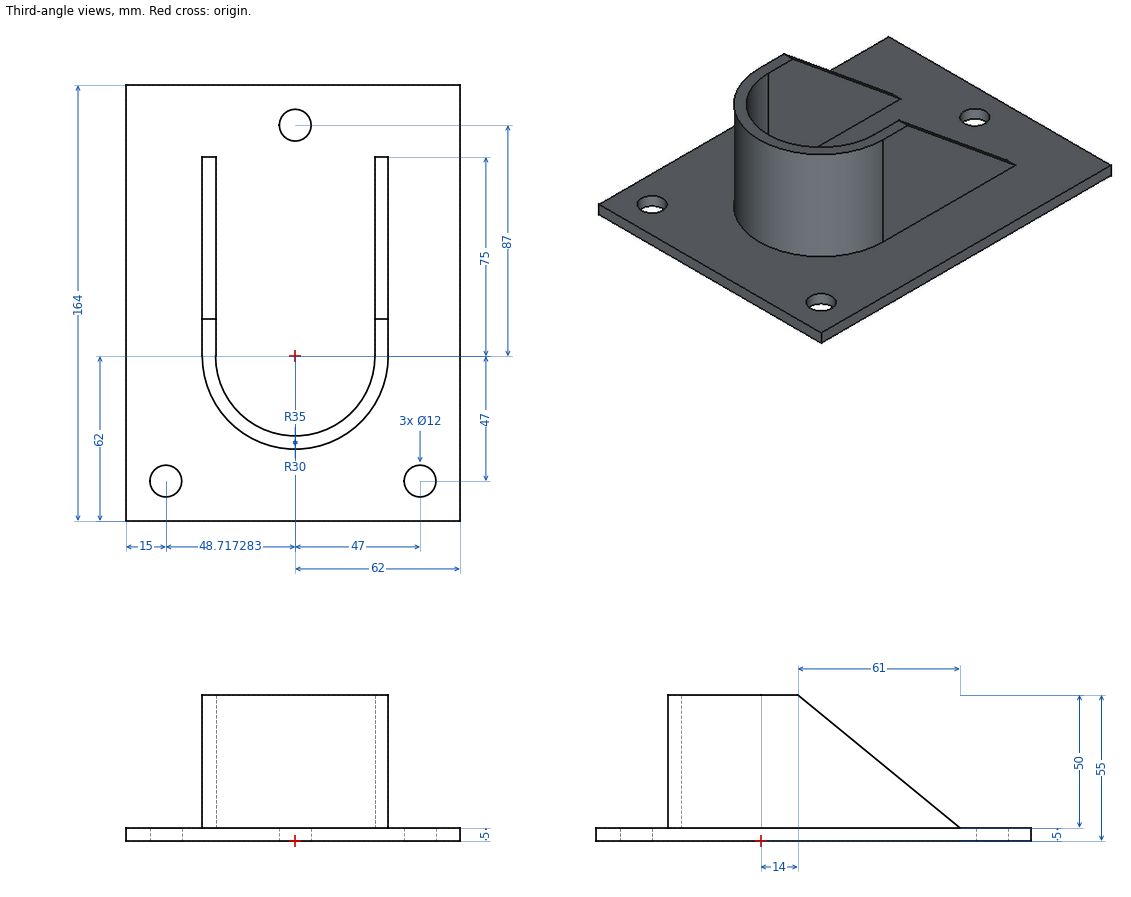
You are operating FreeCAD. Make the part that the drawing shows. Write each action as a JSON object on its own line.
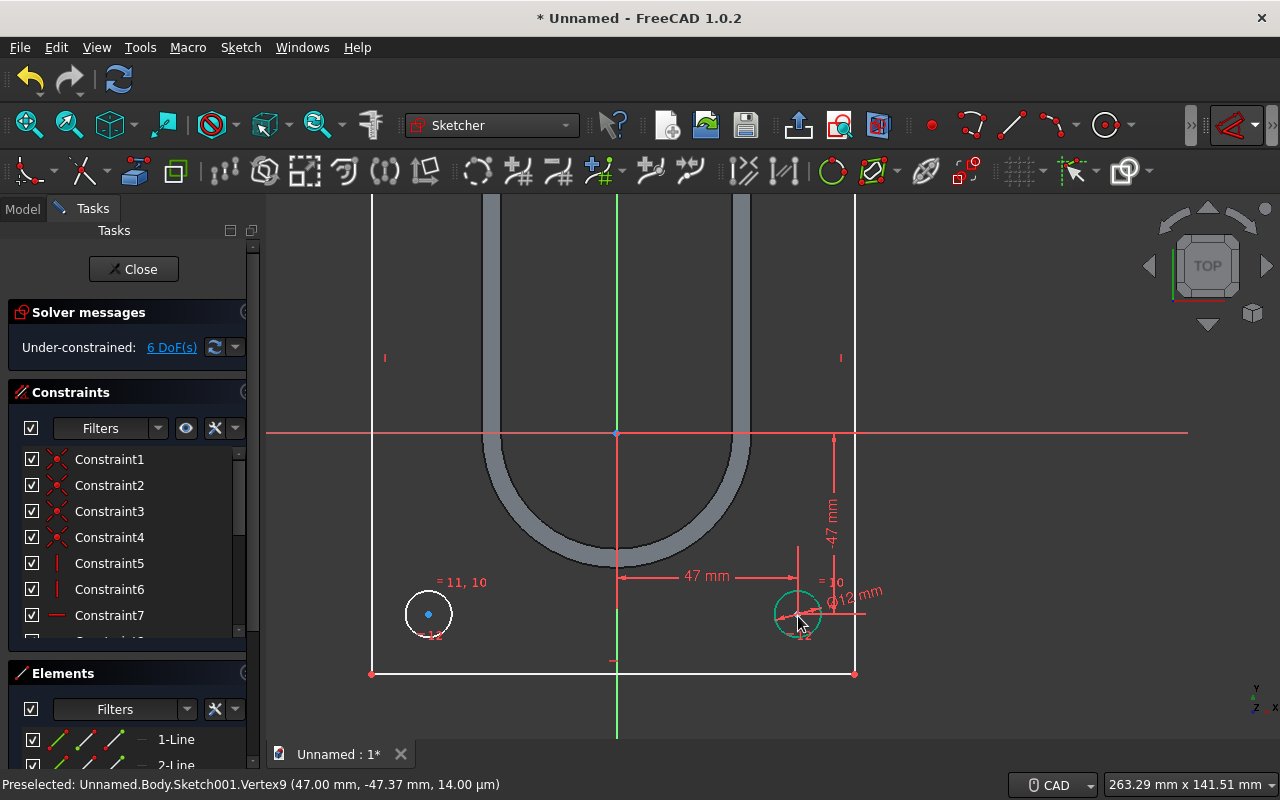
{"action": "scroll", "coordinate": [815, 601], "scroll_direction": "down", "scroll_amount": 3}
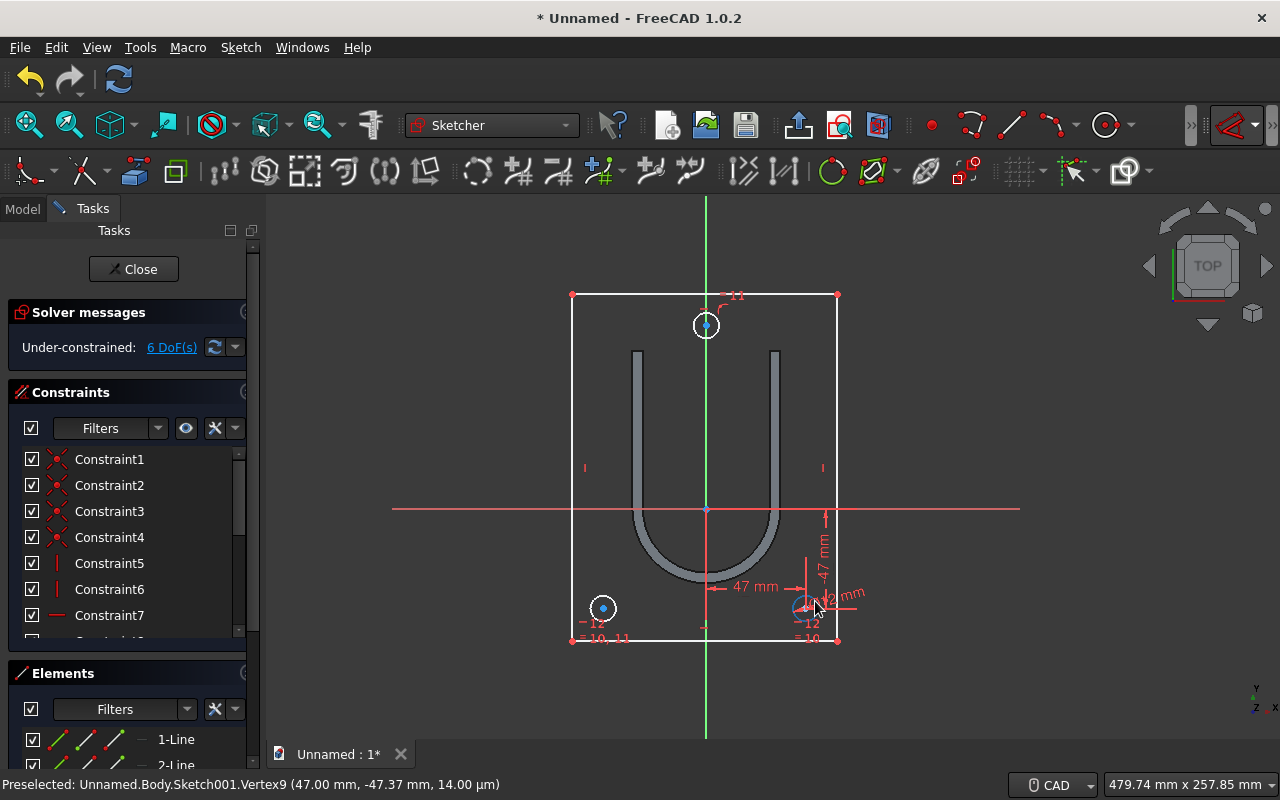
{"action": "left_click", "coordinate": [706, 326]}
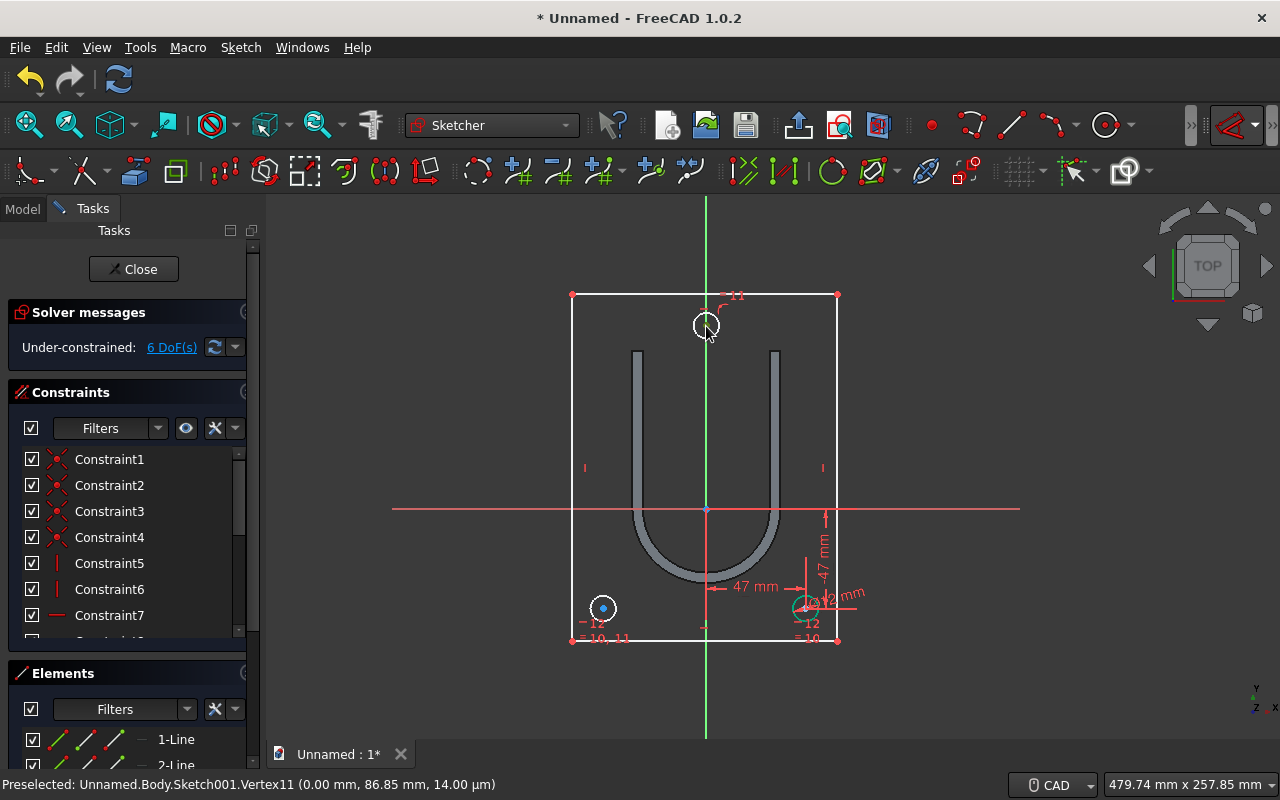
{"action": "left_click", "coordinate": [1258, 126]}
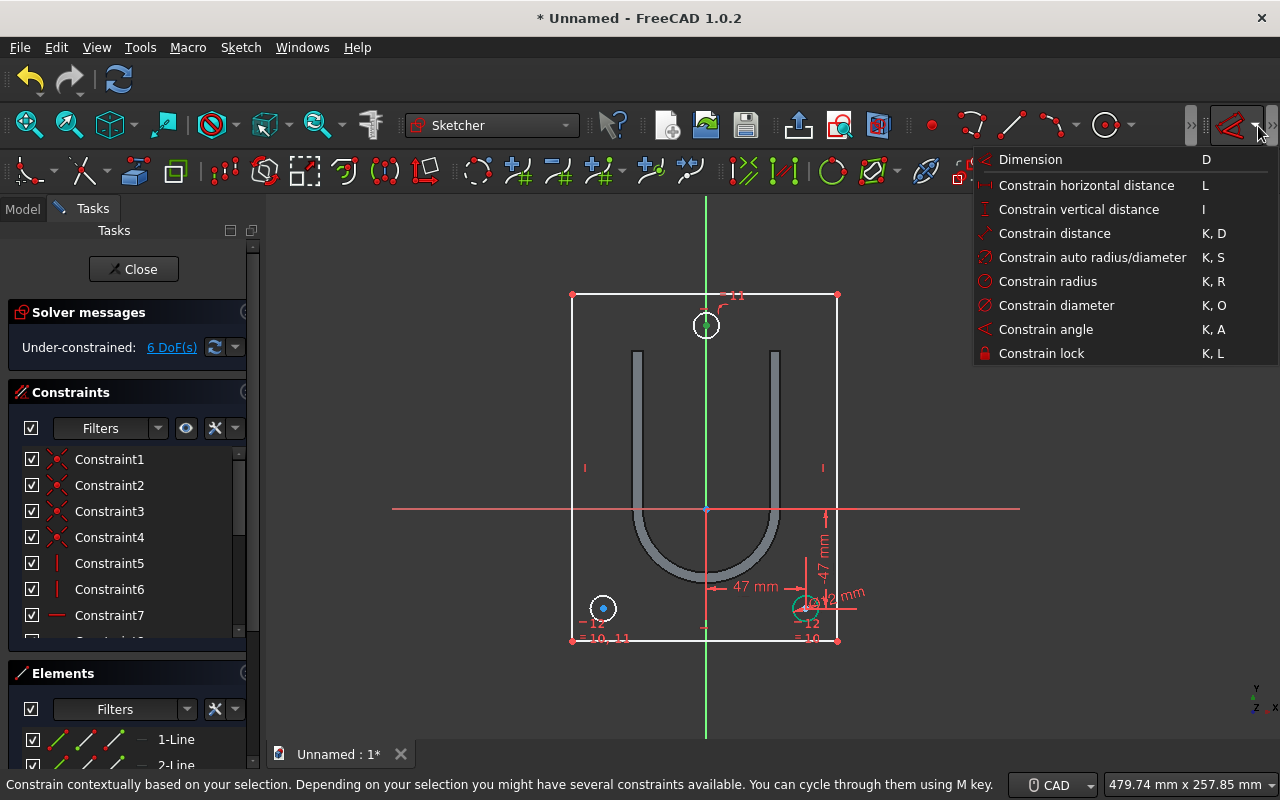
{"action": "left_click", "coordinate": [1126, 209]}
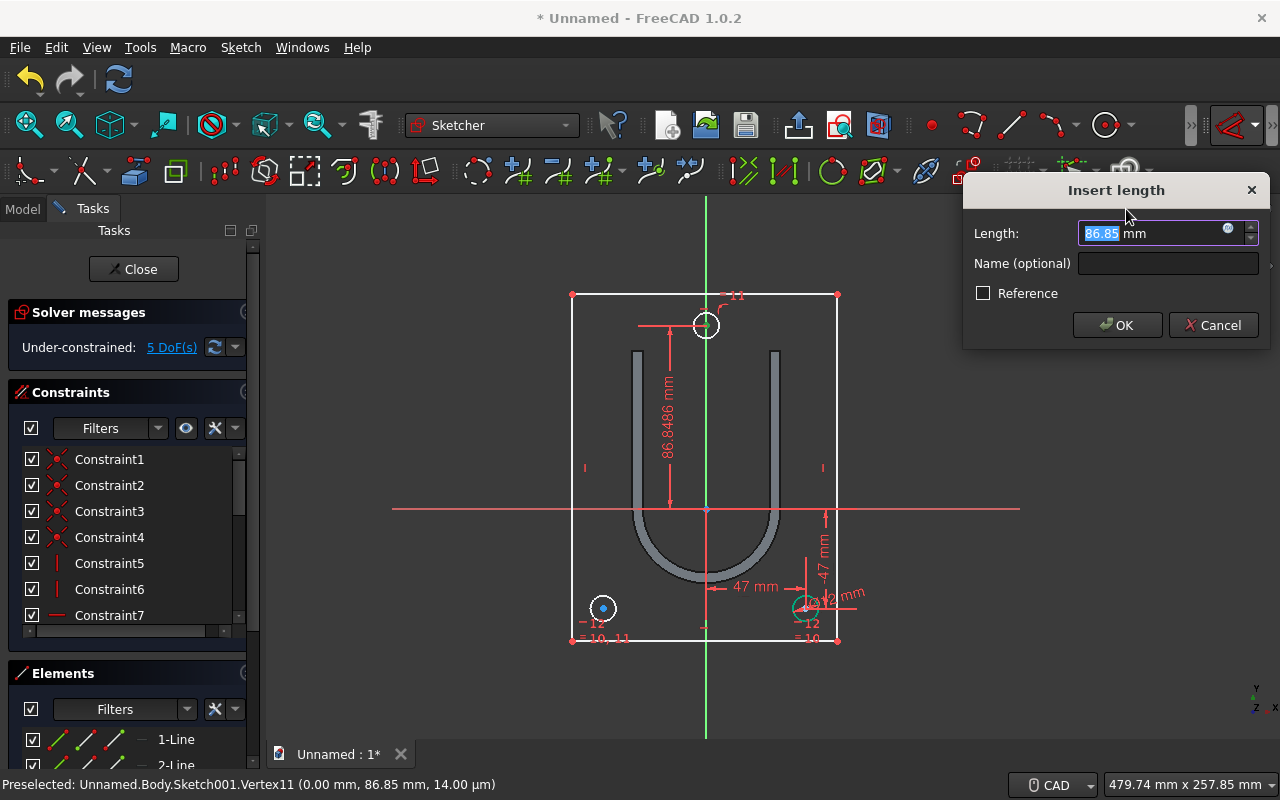
{"action": "type", "text": "87"}
{"action": "key", "text": "Return"}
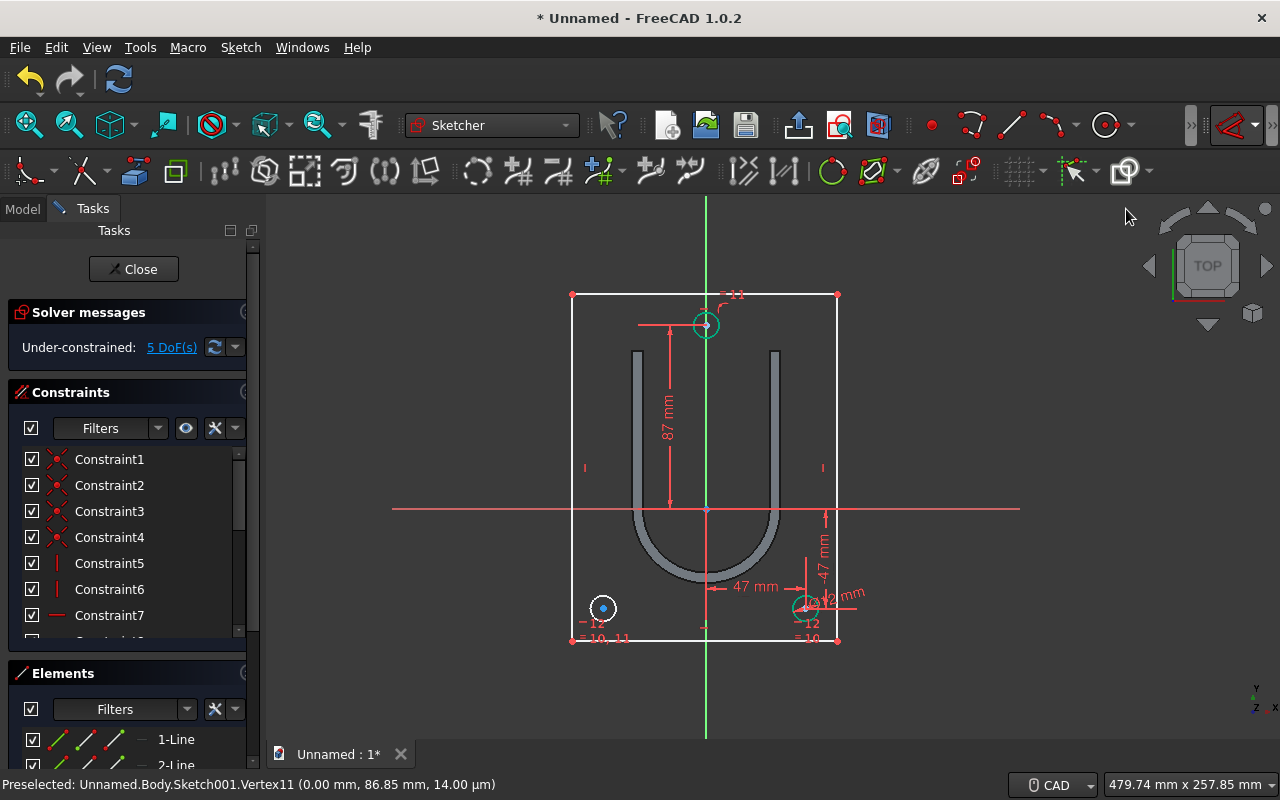
{"action": "left_click", "coordinate": [572, 399]}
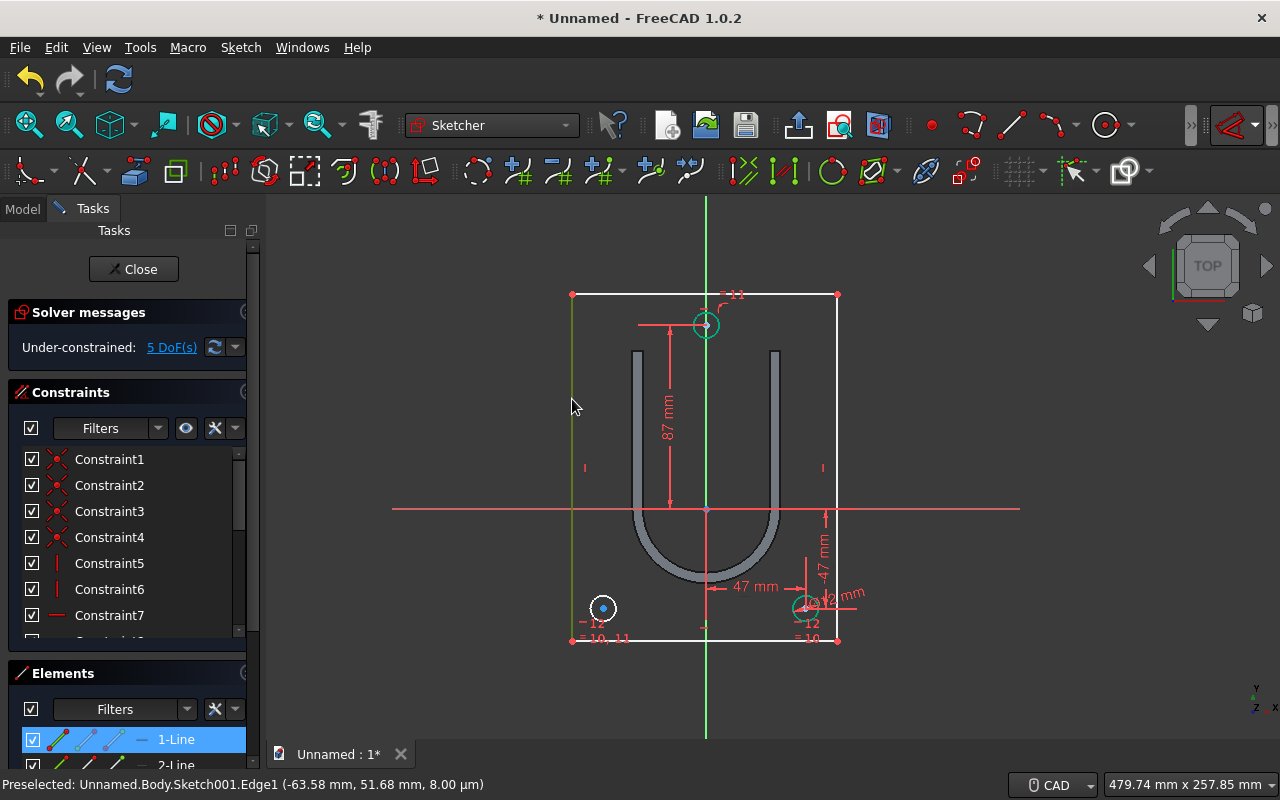
{"action": "key", "text": "i"}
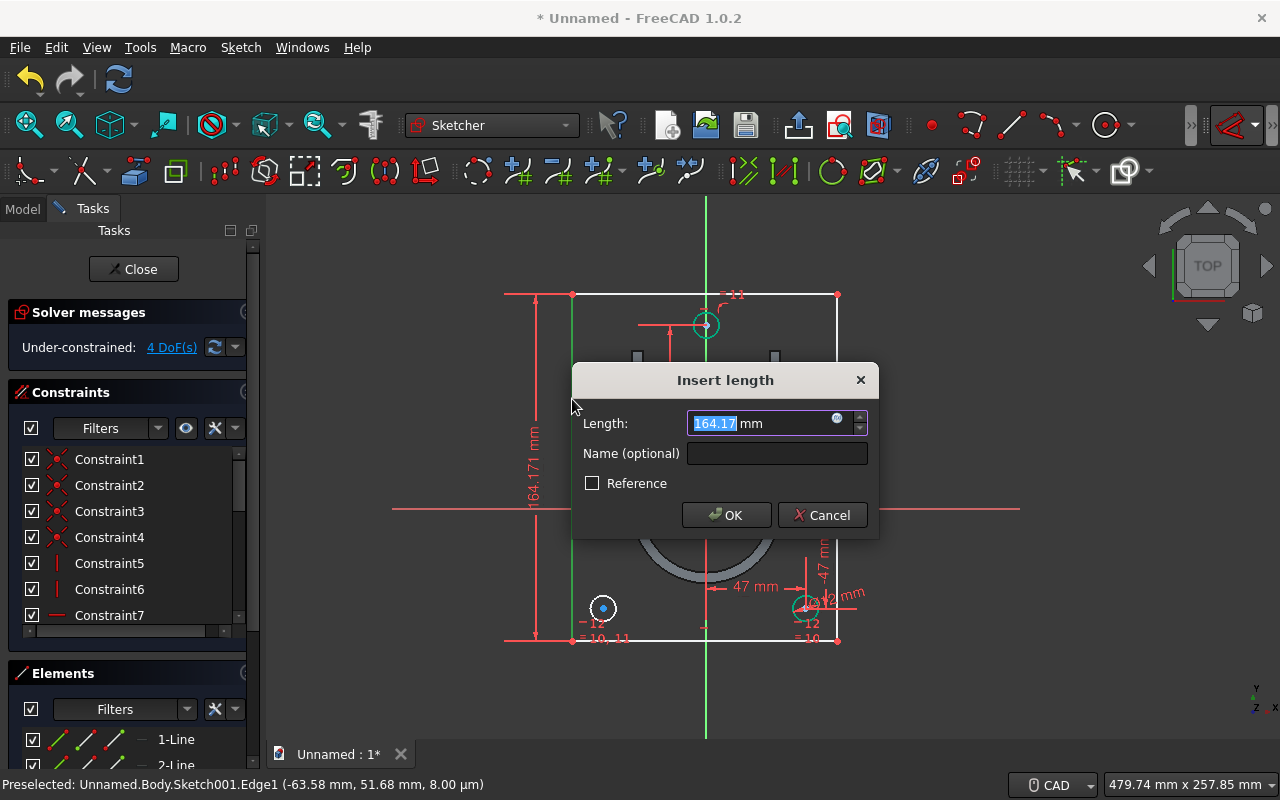
{"action": "type", "text": "164"}
{"action": "key", "text": "Return"}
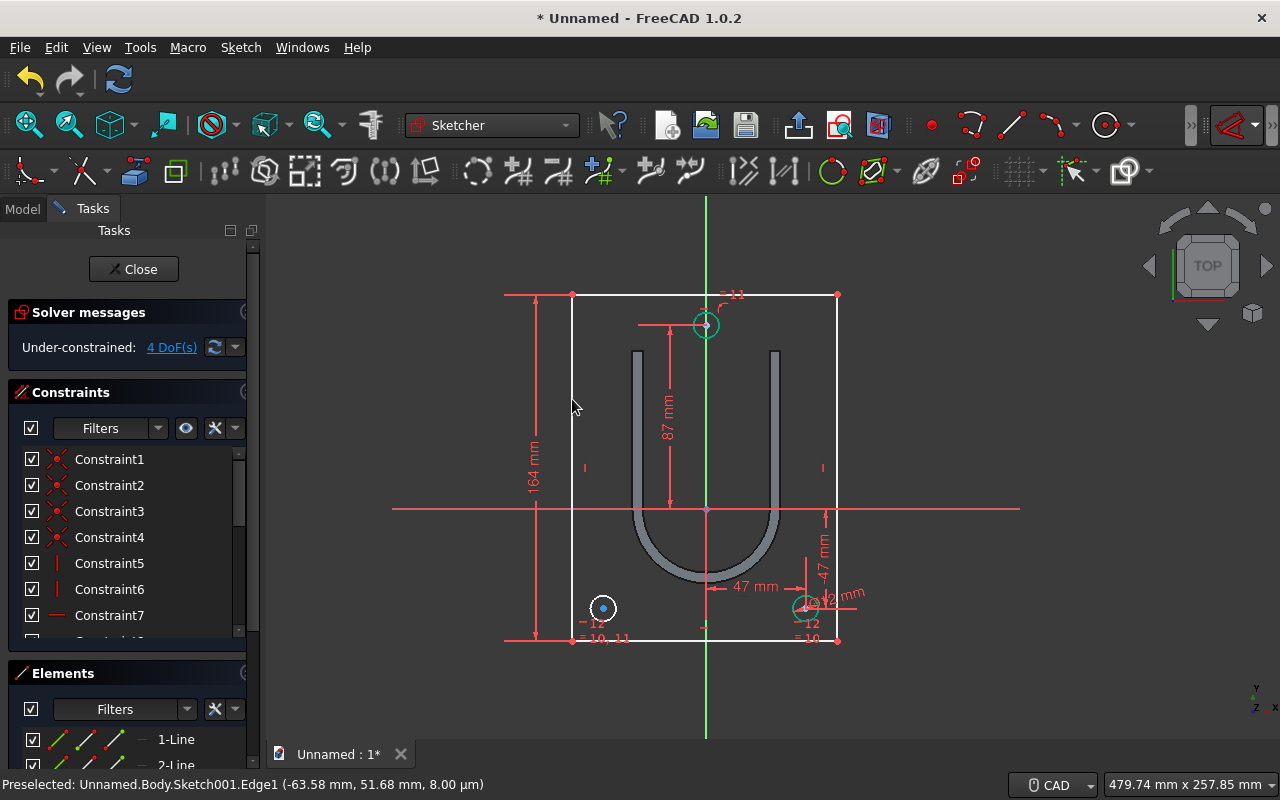
{"action": "left_click", "coordinate": [572, 641]}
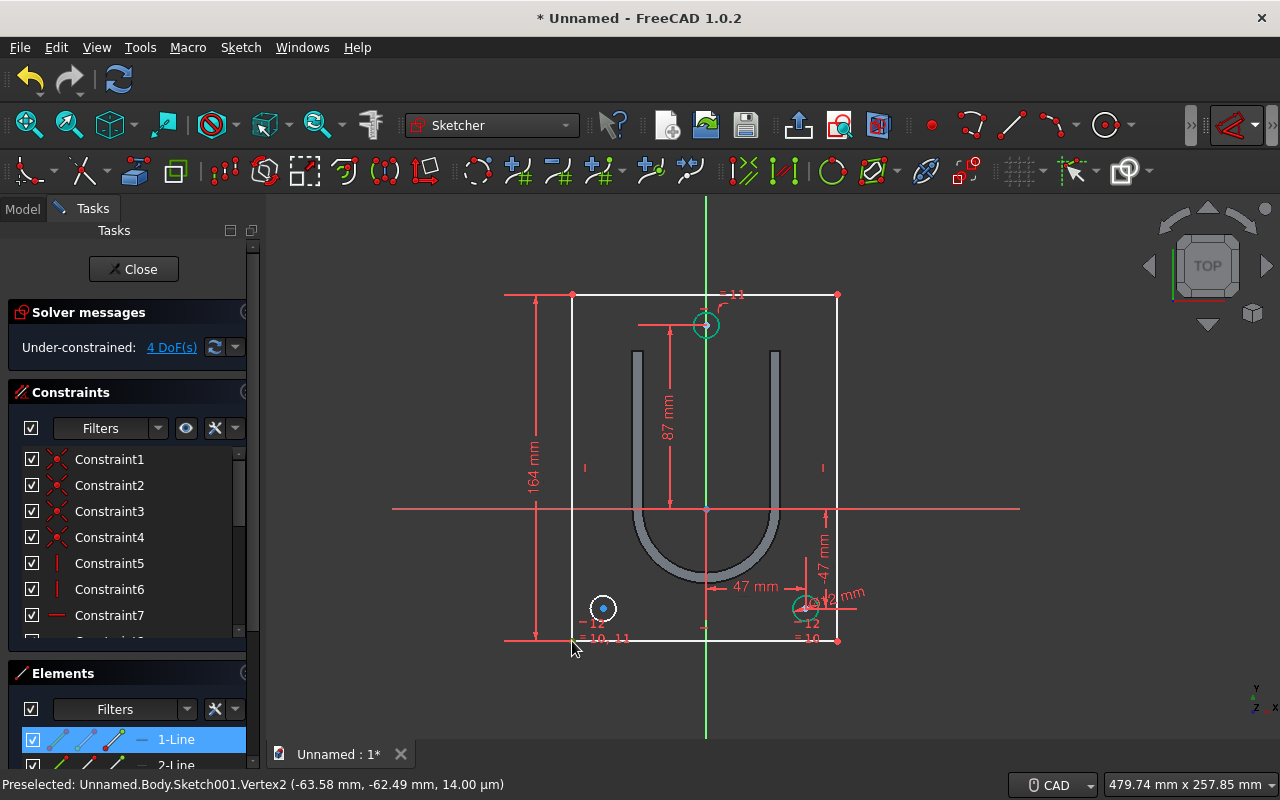
{"action": "key", "text": "i"}